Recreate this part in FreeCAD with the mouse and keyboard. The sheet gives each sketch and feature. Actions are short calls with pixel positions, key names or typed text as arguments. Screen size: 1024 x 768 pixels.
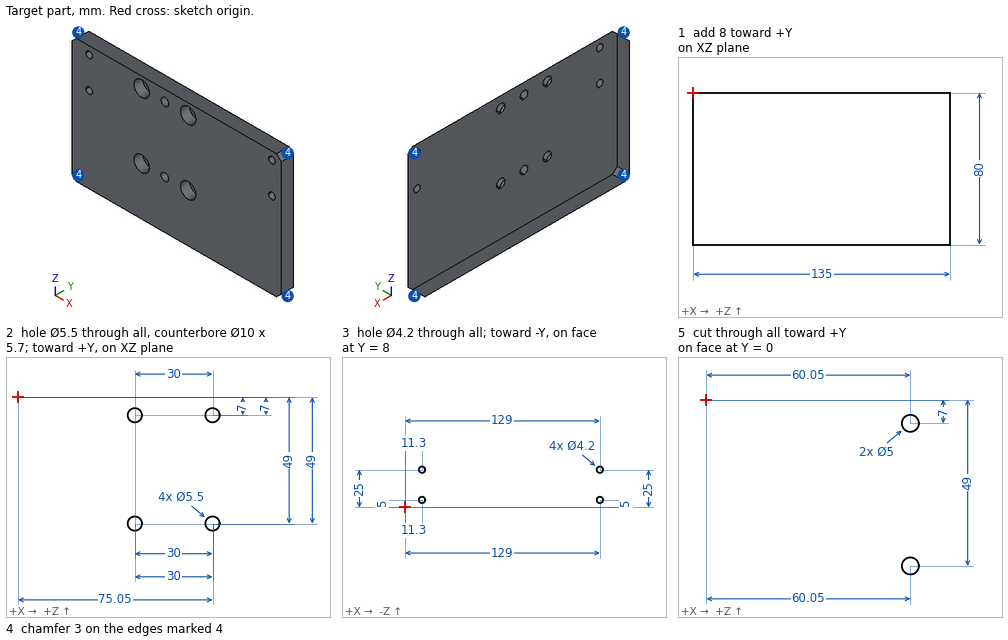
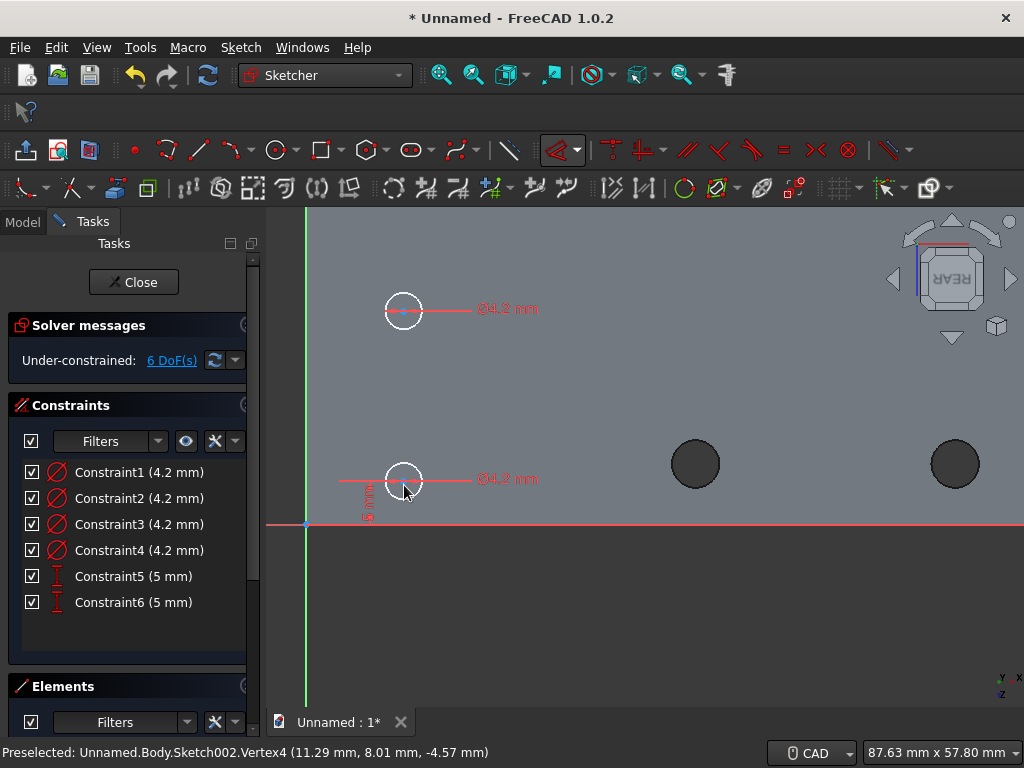
scroll(404, 486, down, 5)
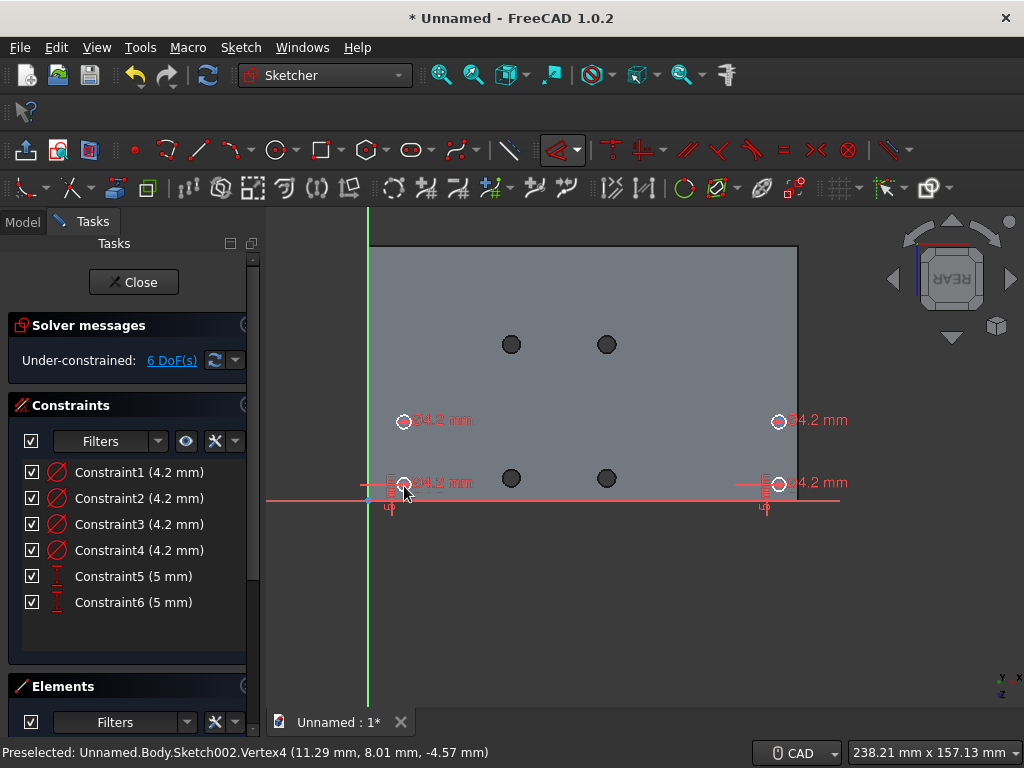
click(779, 422)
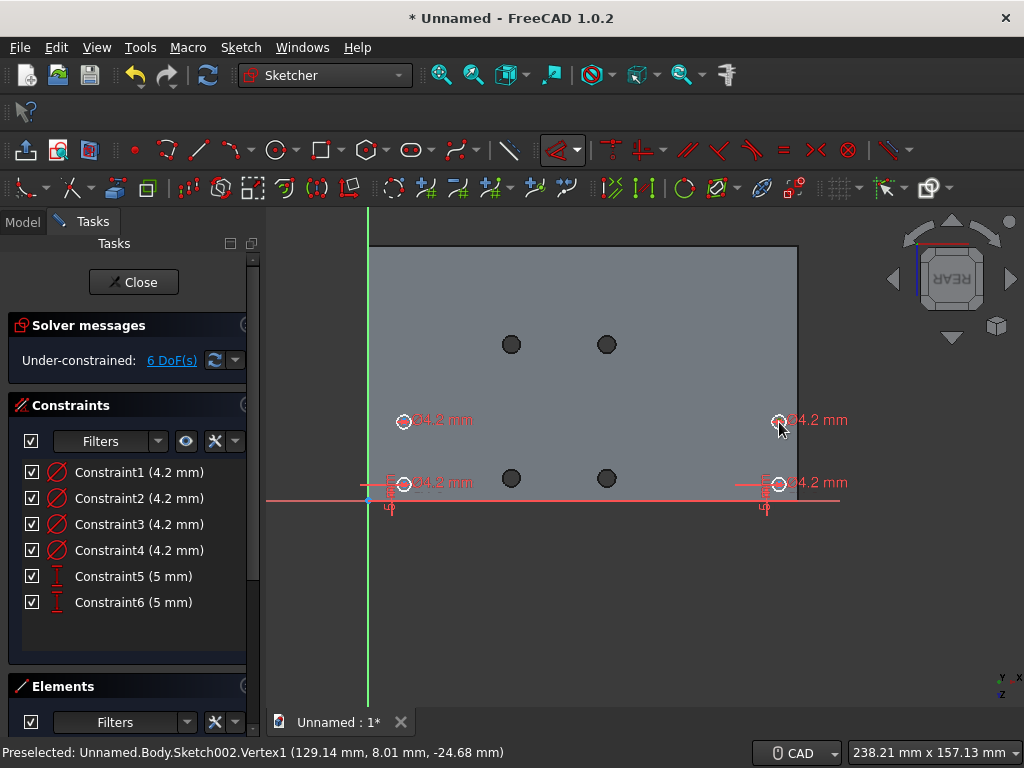
key(i)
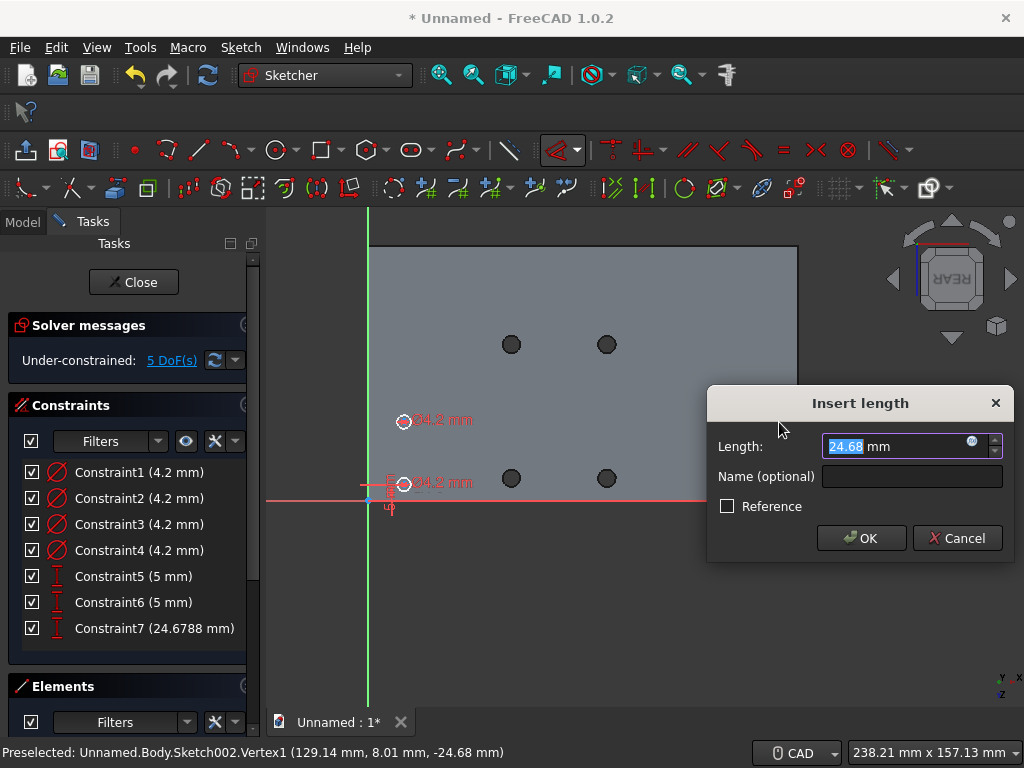
text(25)
key(Return)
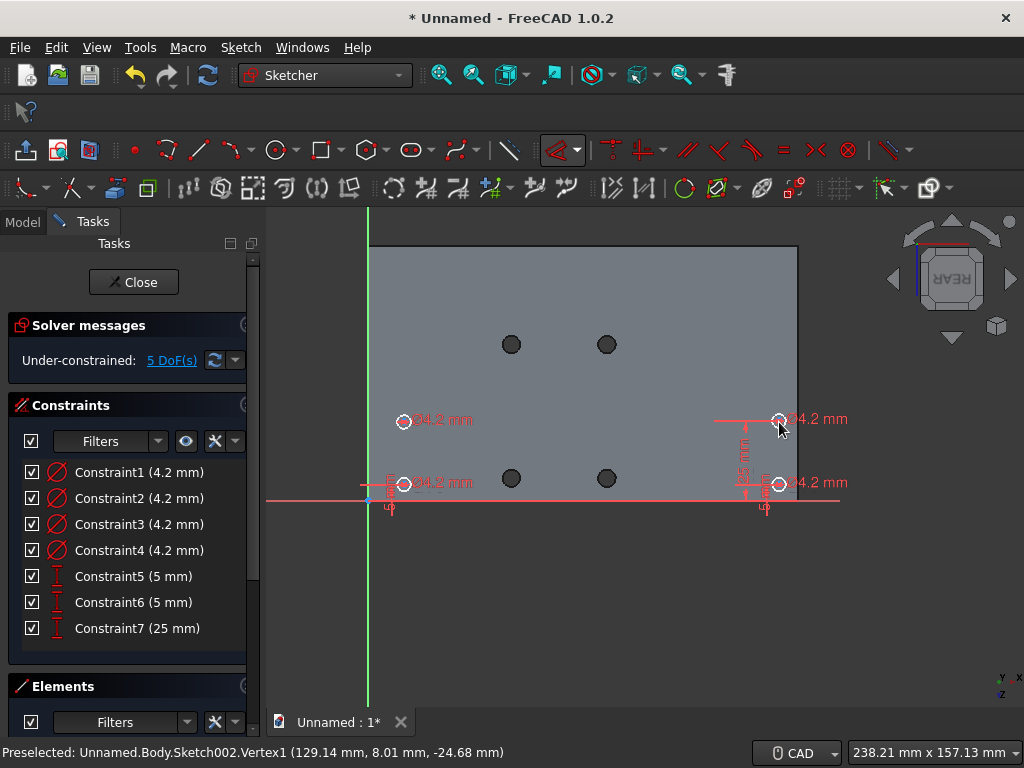
click(404, 422)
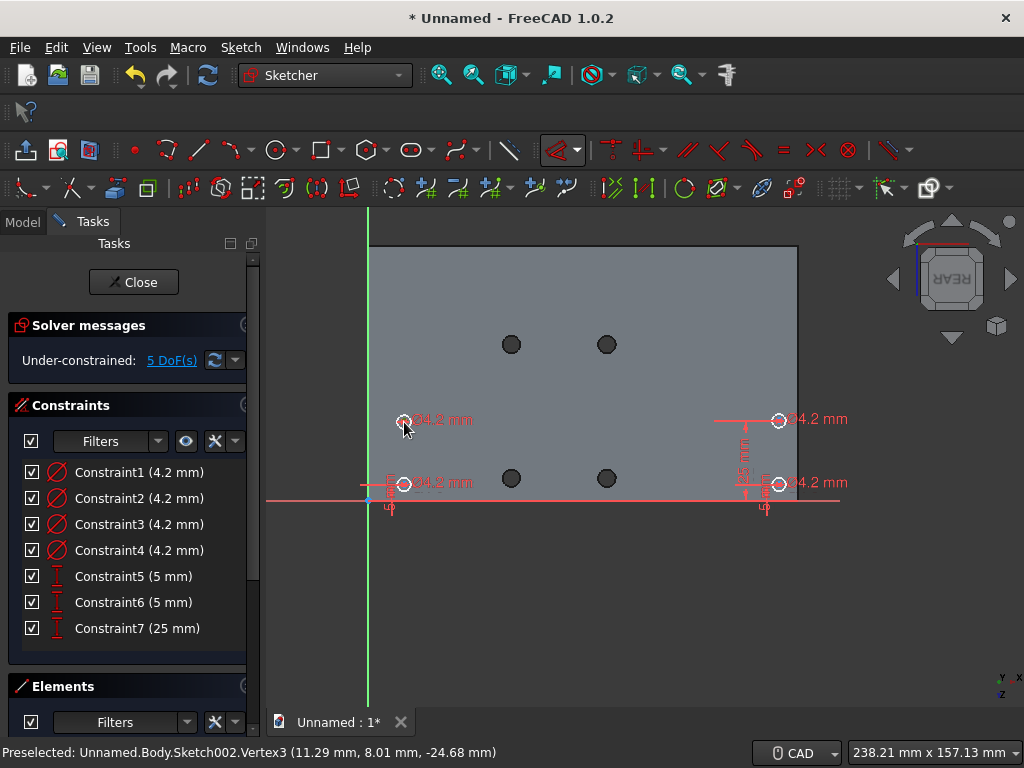
key(i)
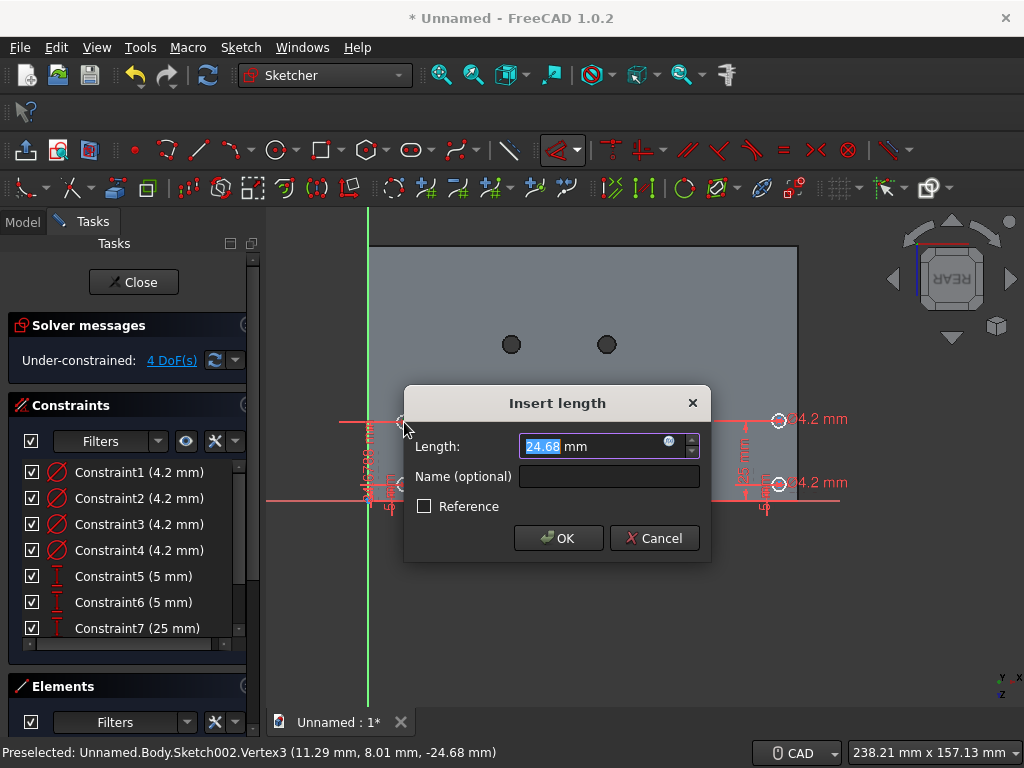
text(25)
key(Return)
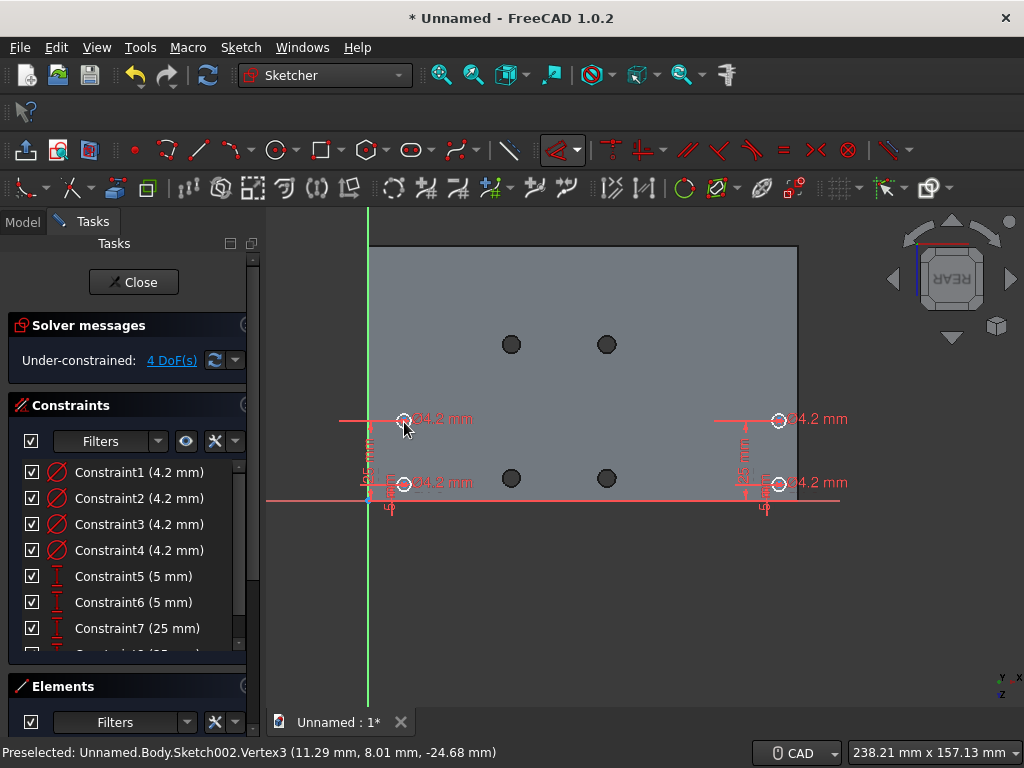
click(779, 421)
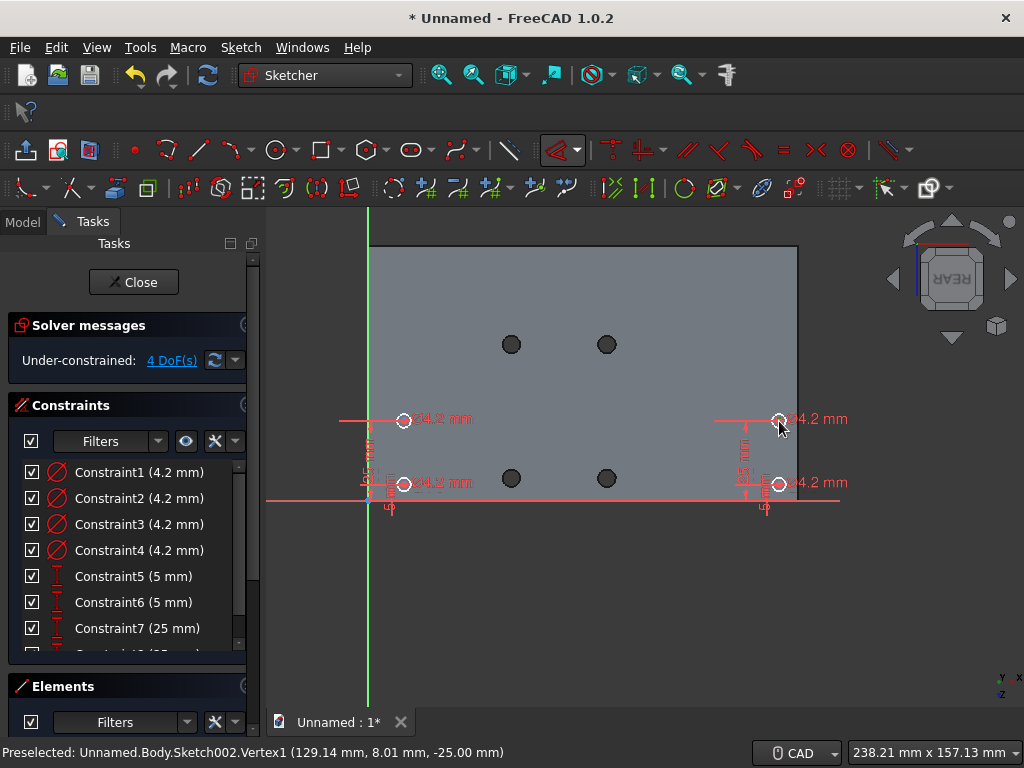
key(l)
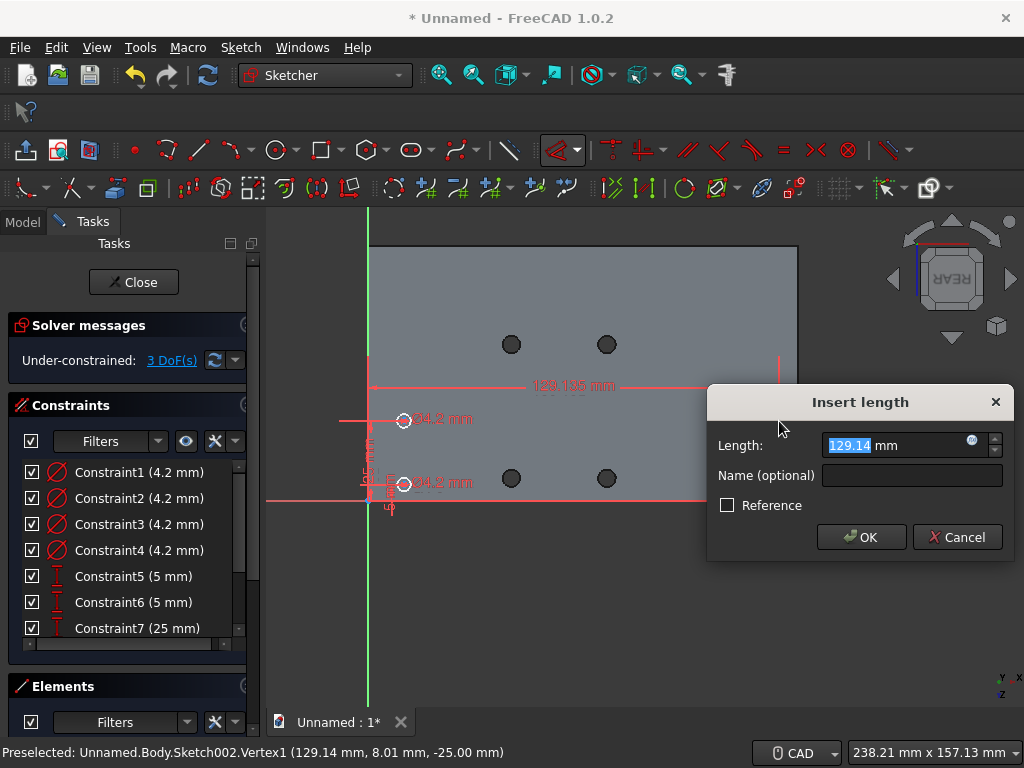
text(129)
key(Return)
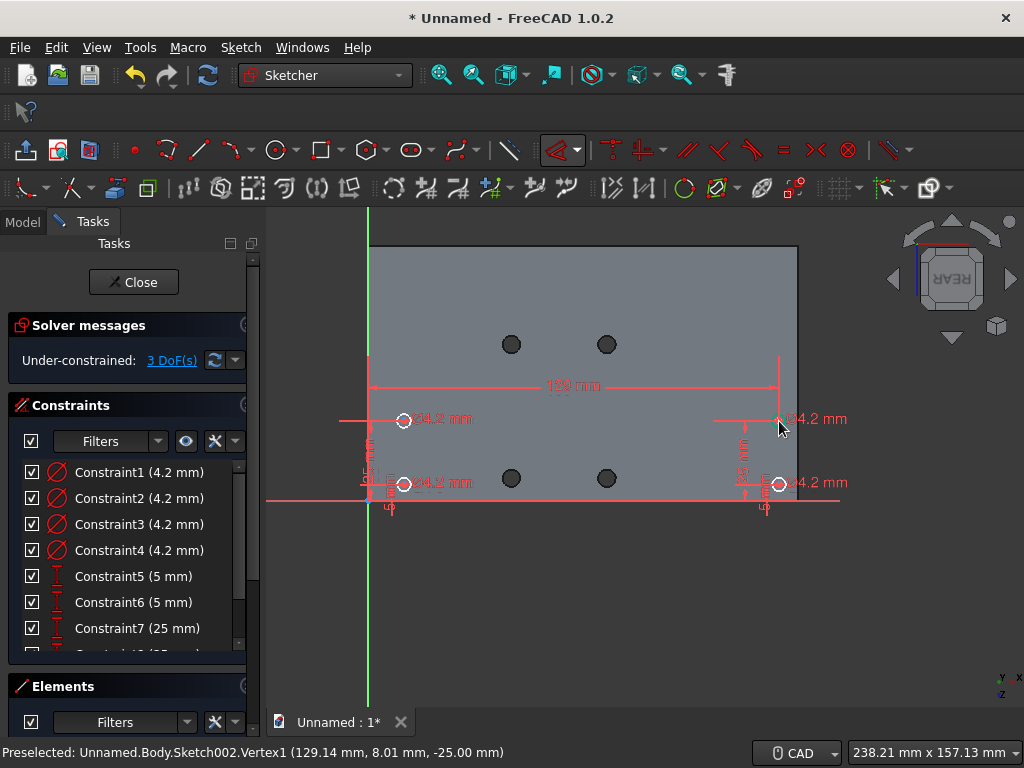
click(779, 485)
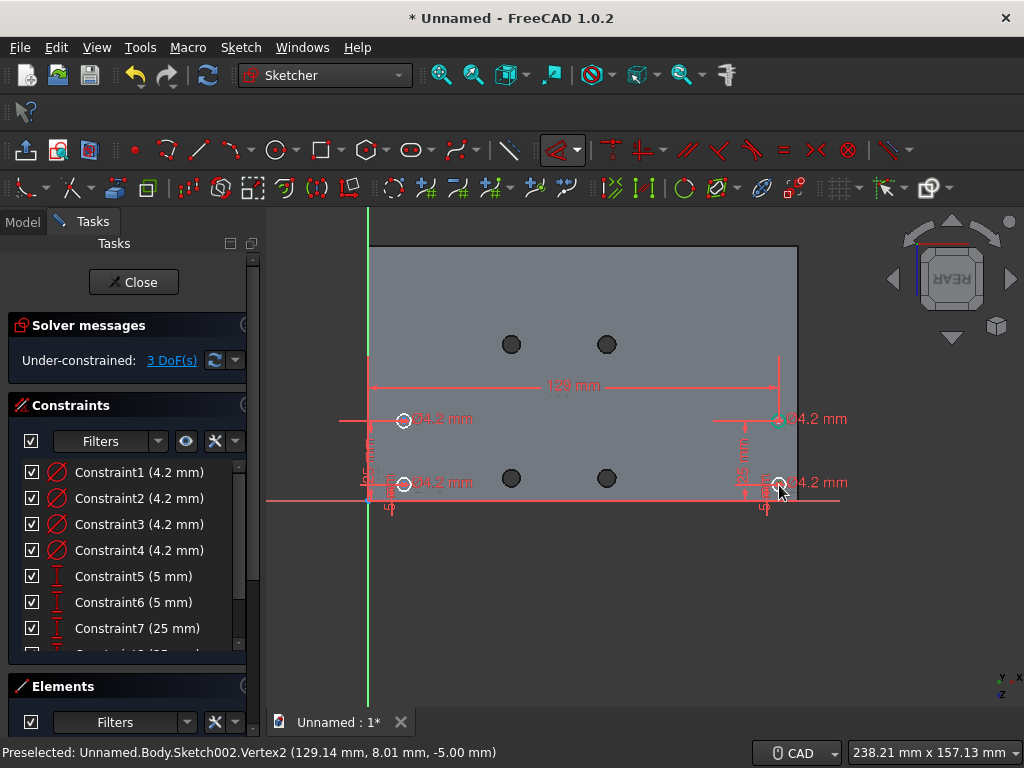
key(l)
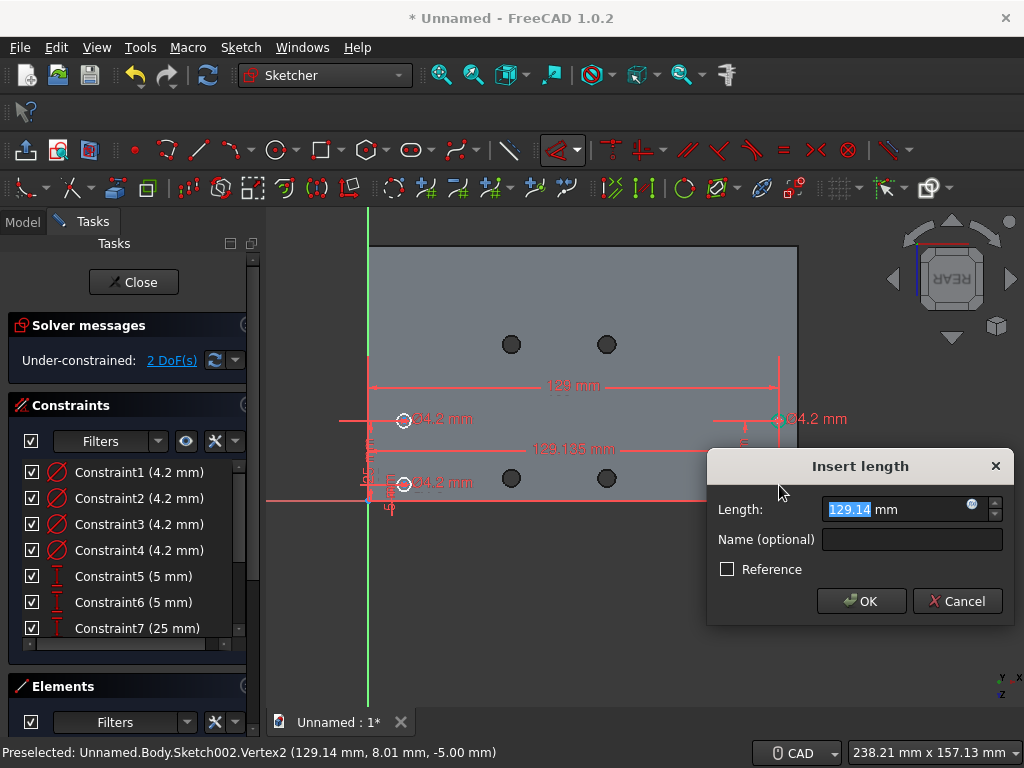
text(129)
key(Return)